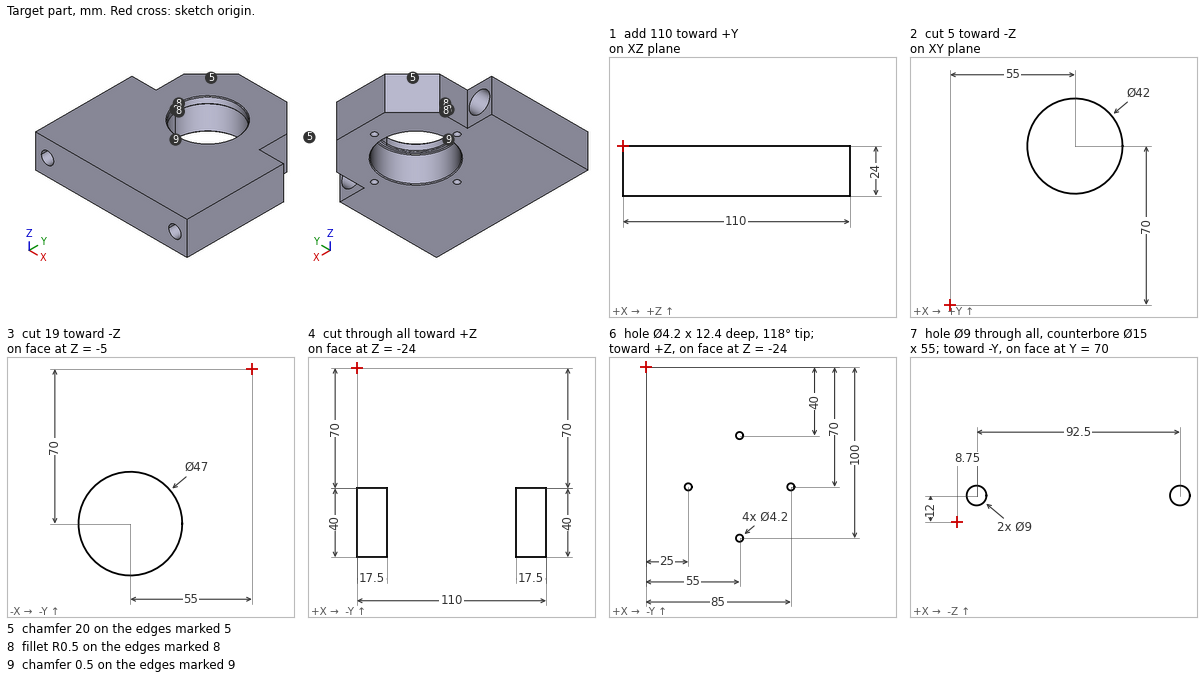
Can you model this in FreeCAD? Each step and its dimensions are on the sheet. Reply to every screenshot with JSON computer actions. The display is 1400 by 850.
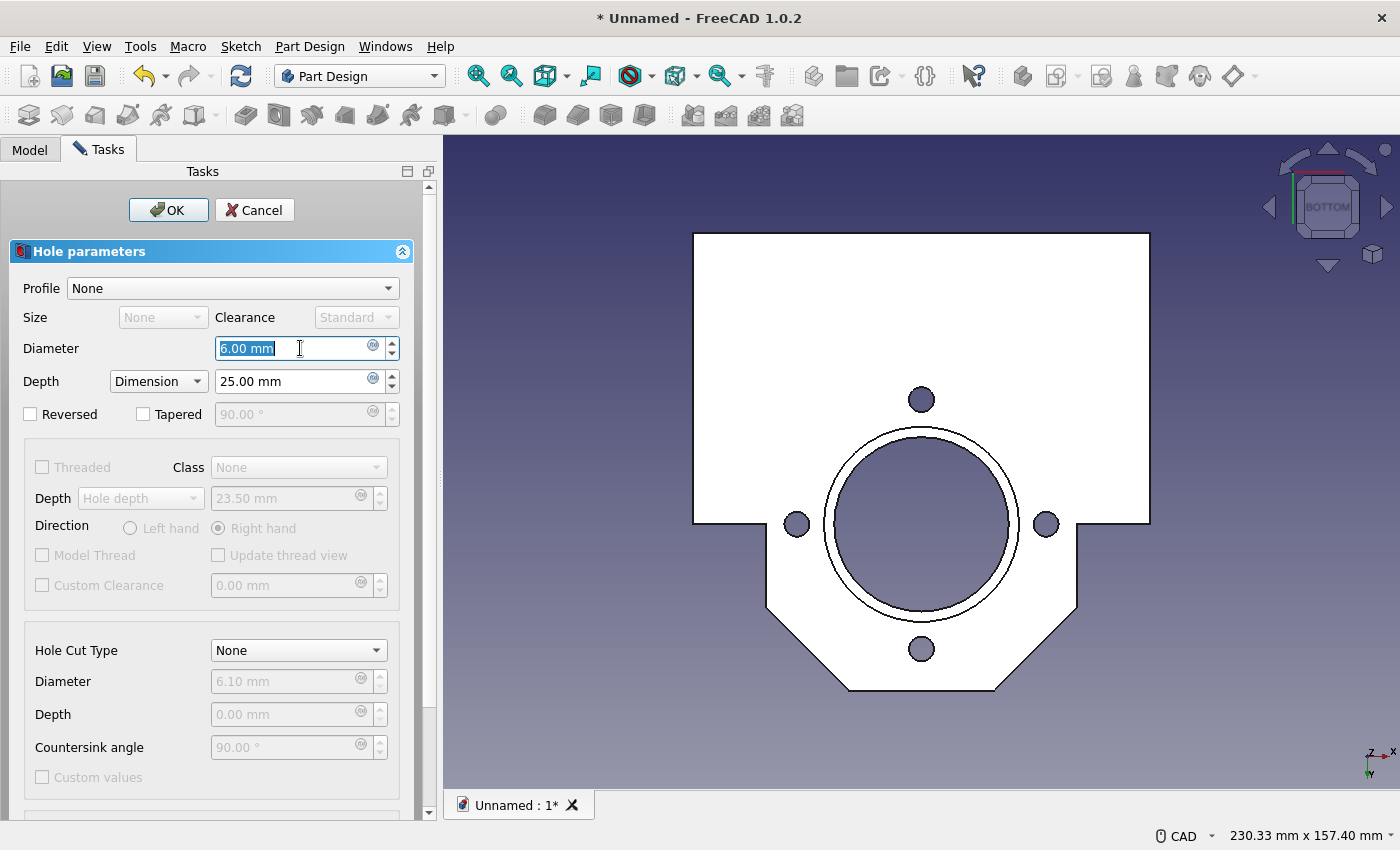
{"action": "type", "text": "4.2"}
{"action": "key", "text": "Tab"}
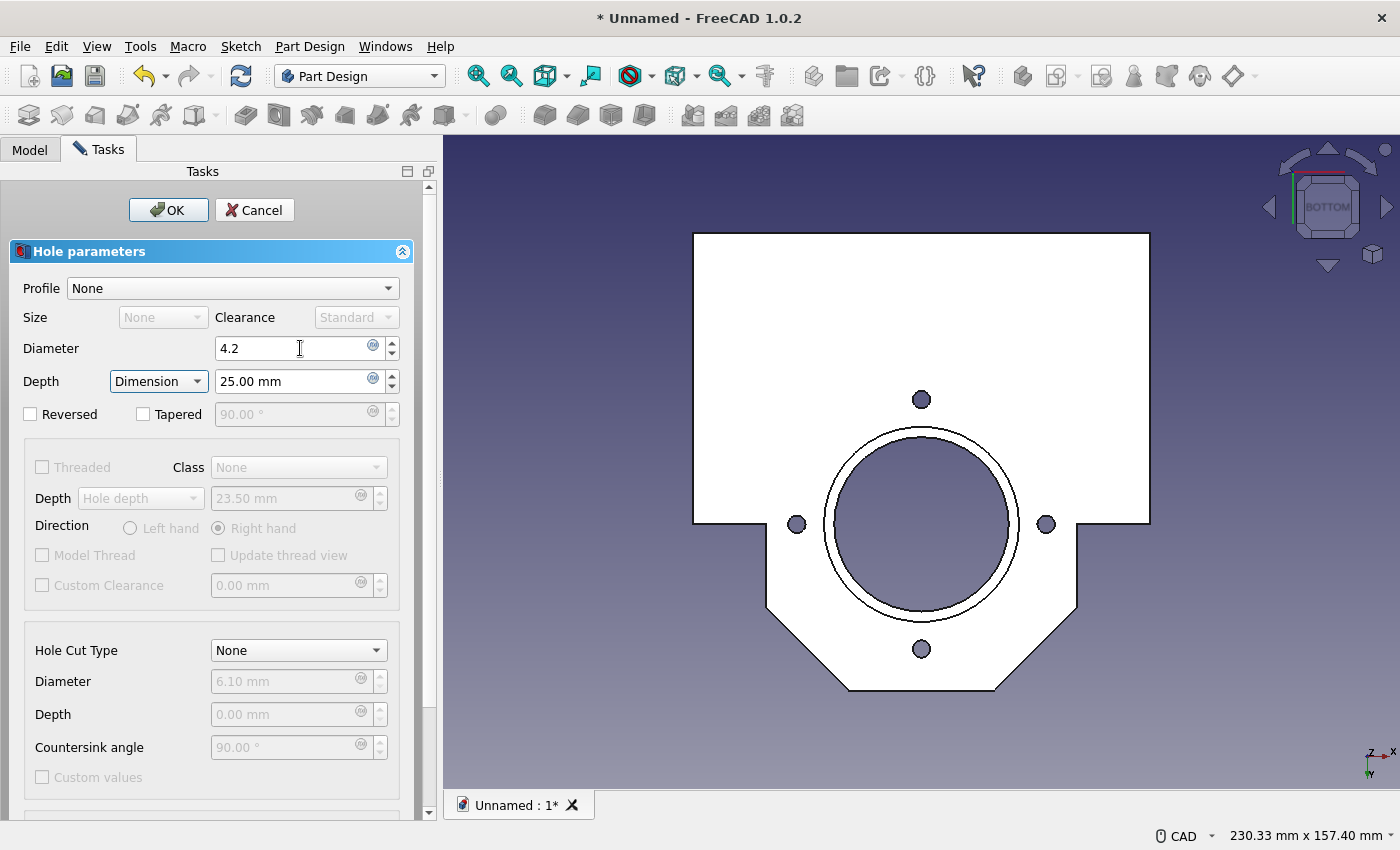
{"action": "triple_click", "coordinate": [300, 382]}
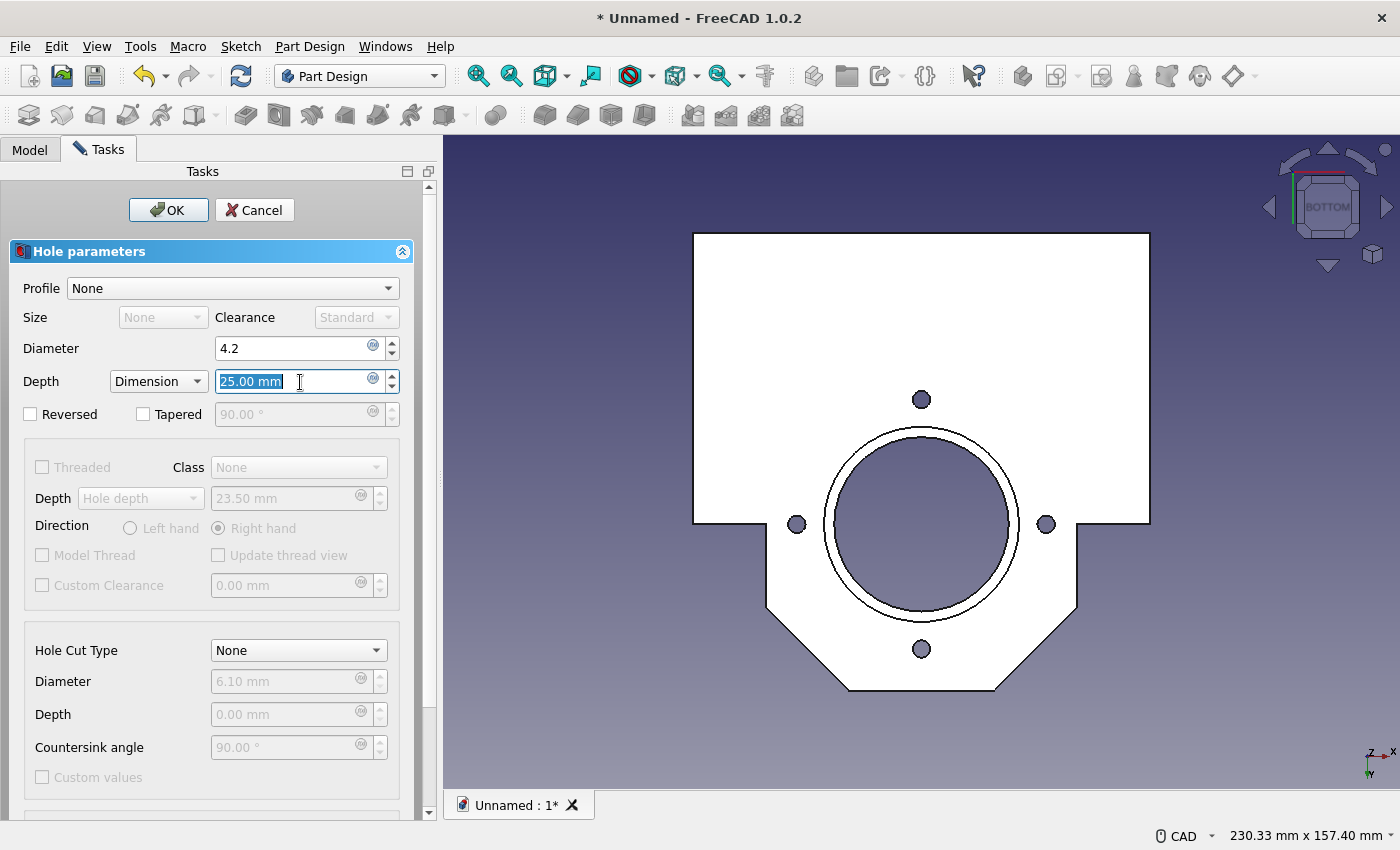
{"action": "type", "text": "12.4"}
{"action": "key", "text": "Tab"}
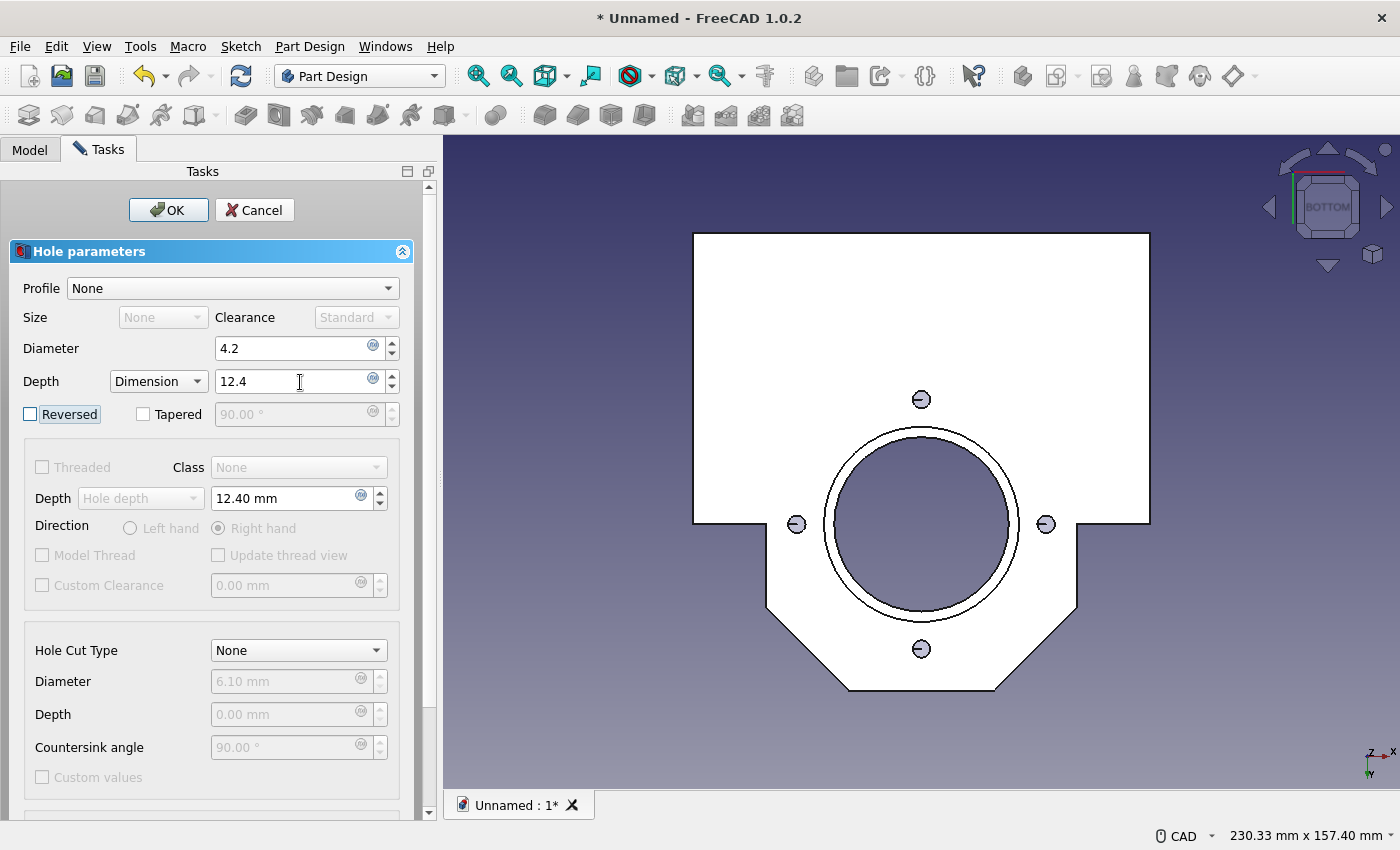
{"action": "left_click", "coordinate": [169, 210]}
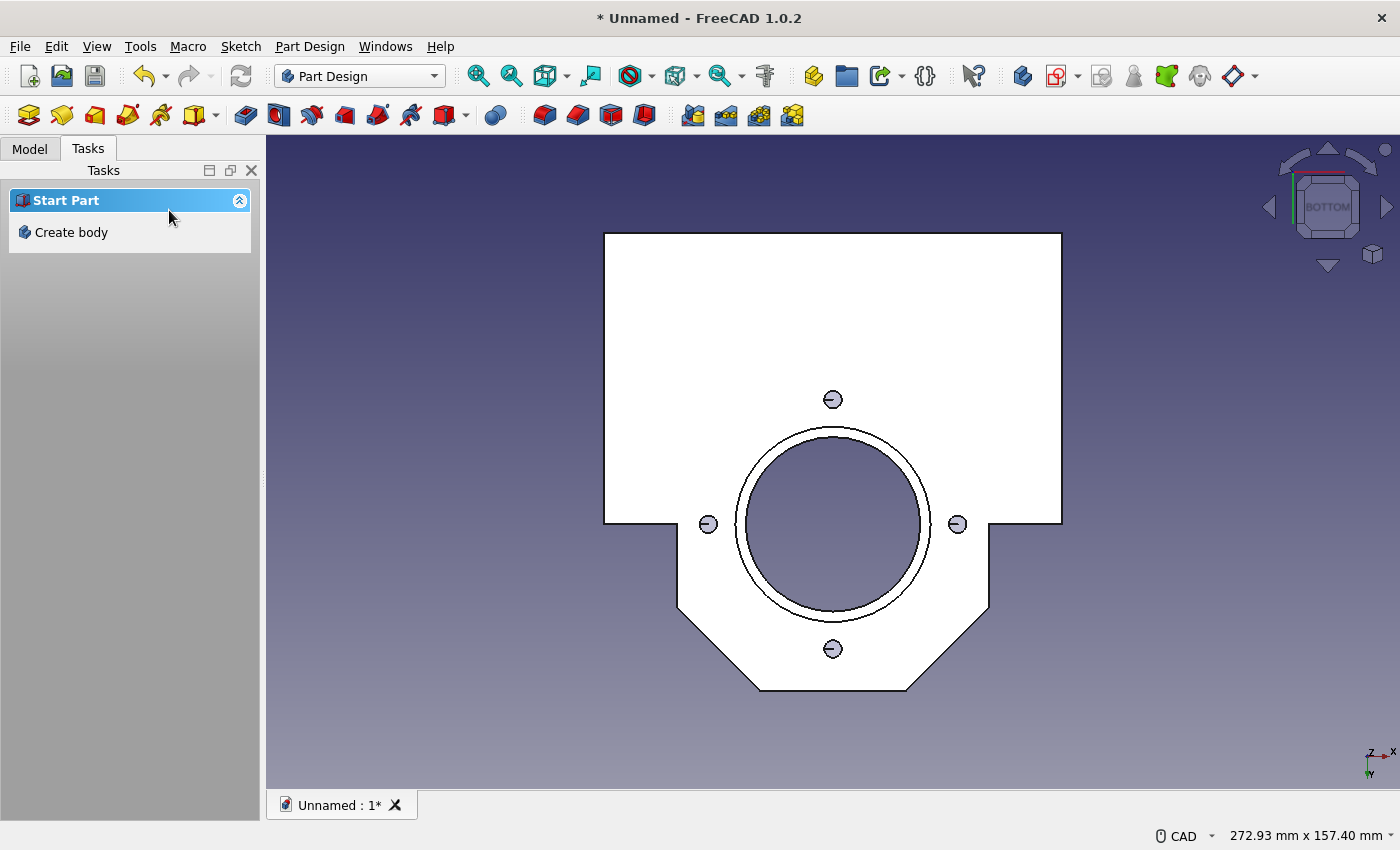
{"action": "key", "text": "4"}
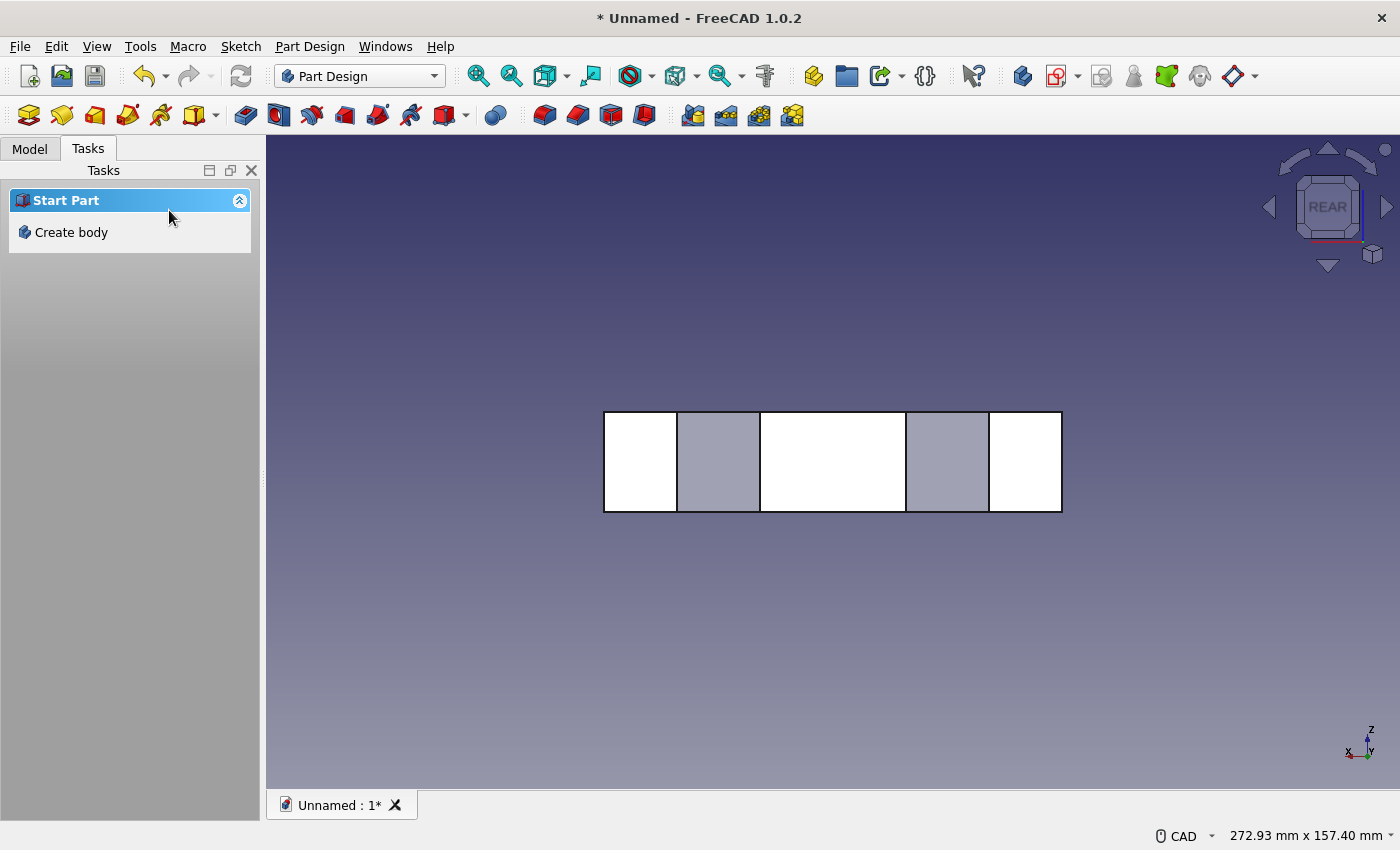
{"action": "left_click", "coordinate": [479, 76]}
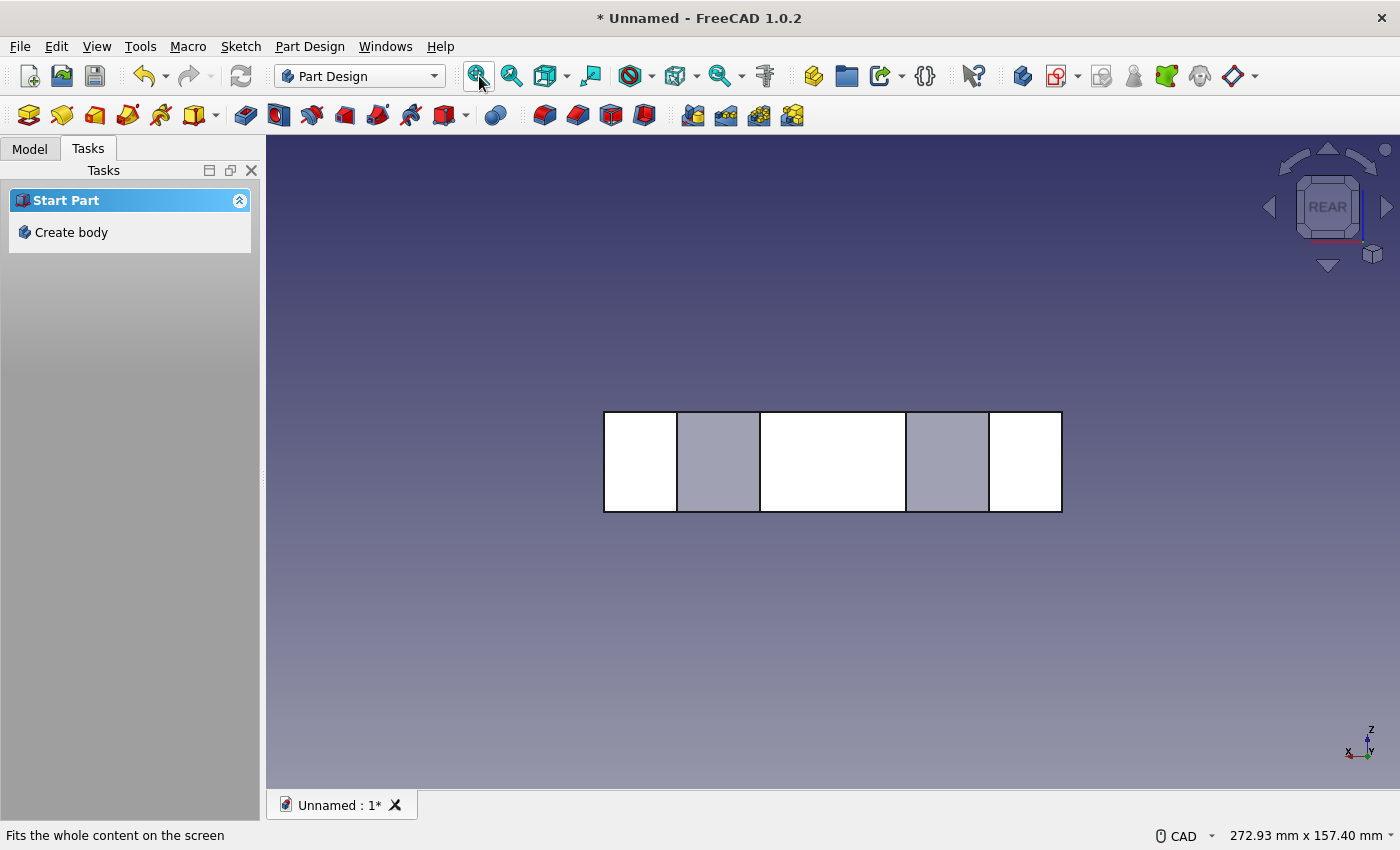
{"action": "left_click", "coordinate": [641, 461]}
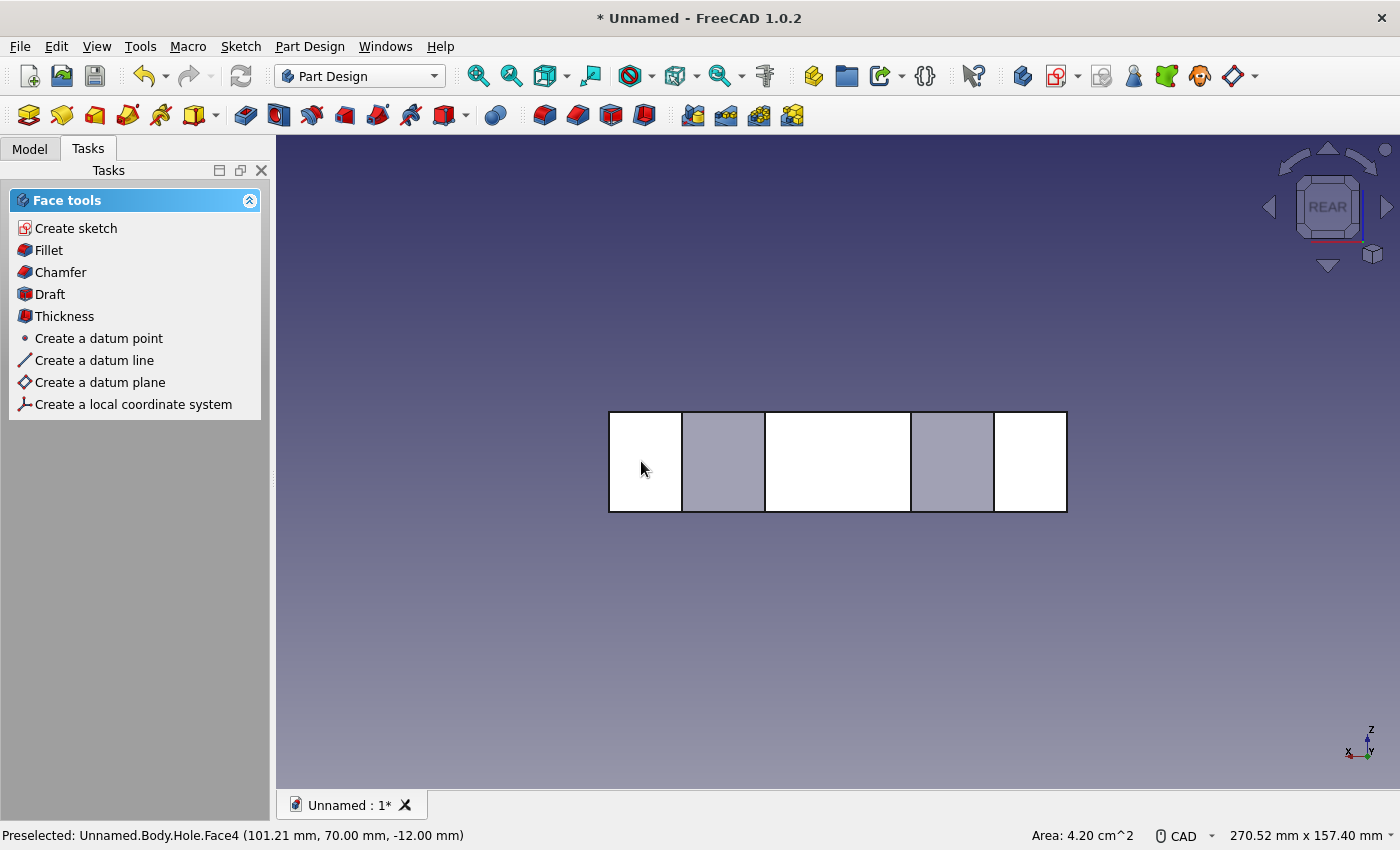
{"action": "left_click", "coordinate": [1056, 76]}